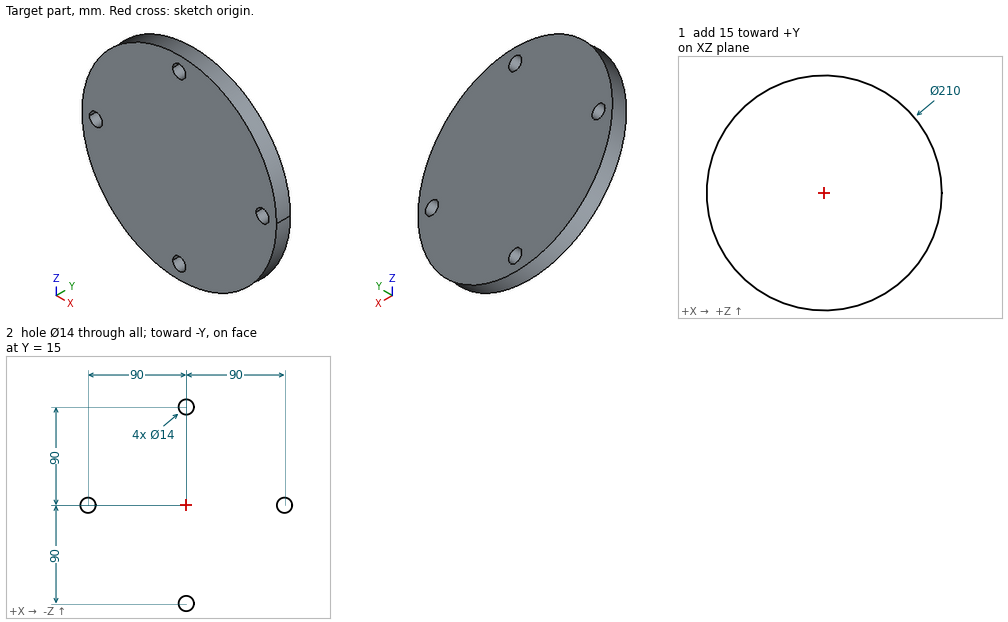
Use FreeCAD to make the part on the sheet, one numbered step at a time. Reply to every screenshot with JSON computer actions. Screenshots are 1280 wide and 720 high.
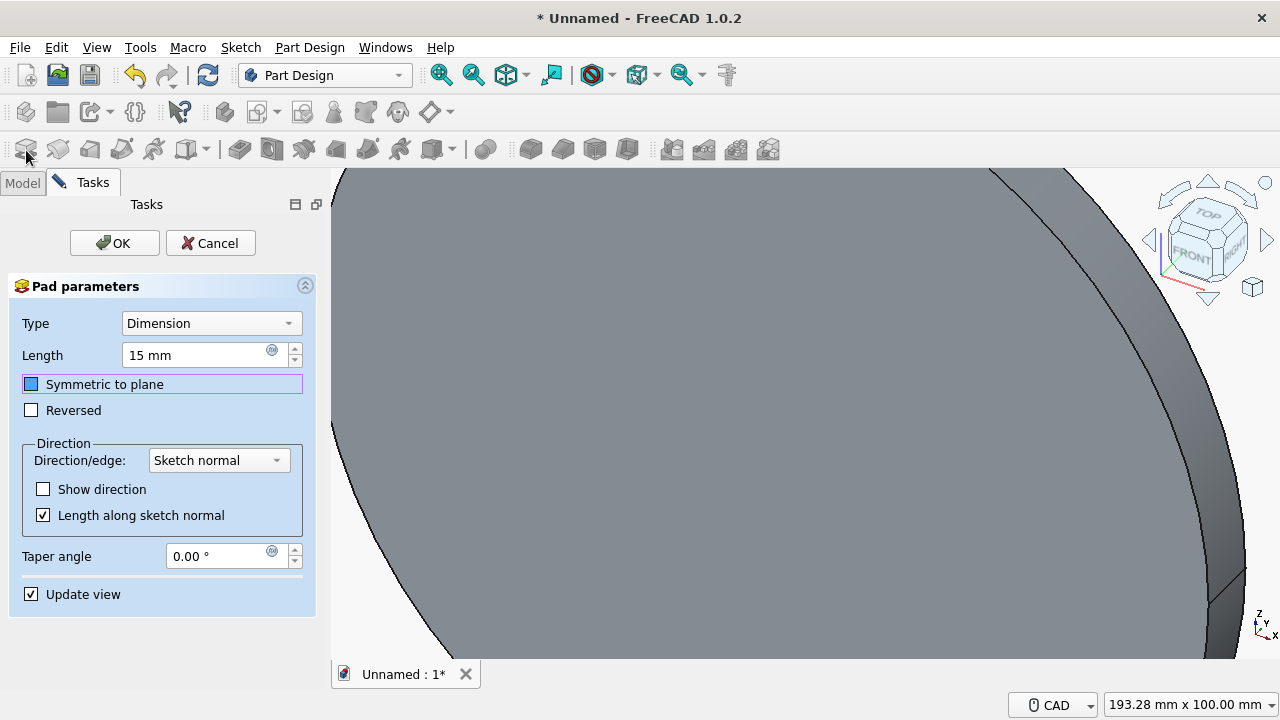
{"action": "left_click", "coordinate": [30, 410]}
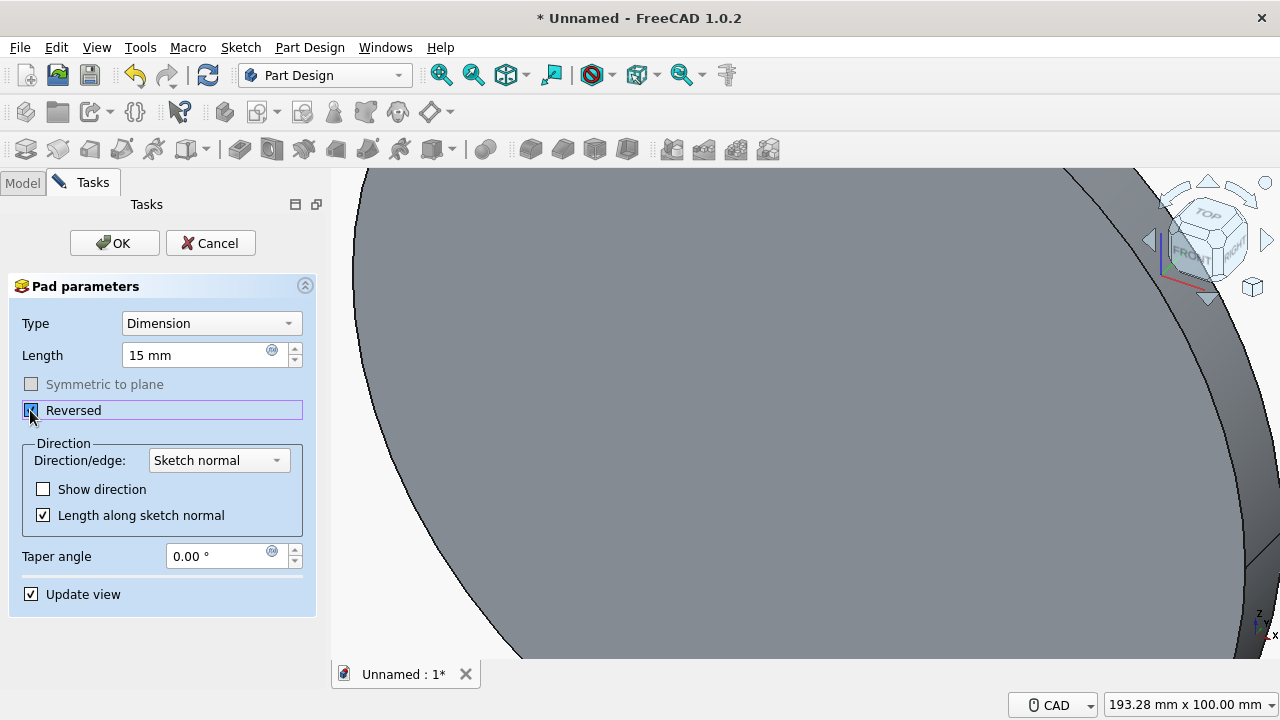
{"action": "left_click", "coordinate": [115, 243]}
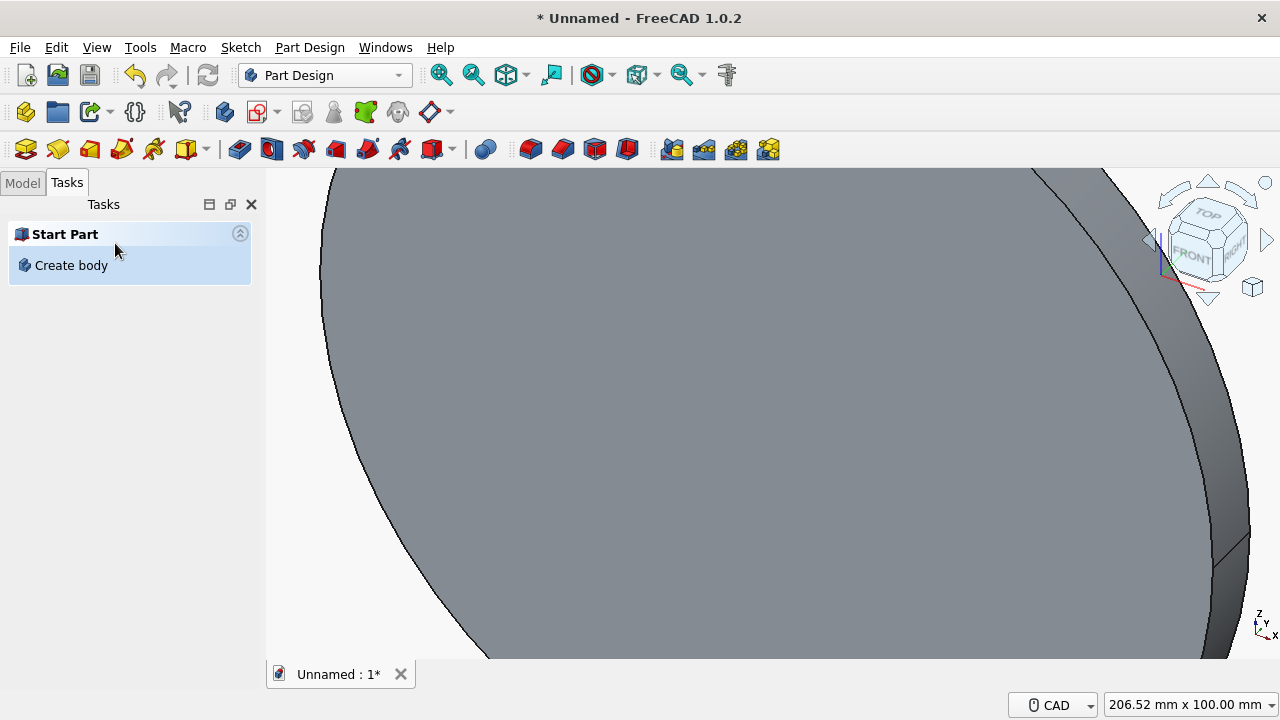
{"action": "left_click", "coordinate": [442, 76]}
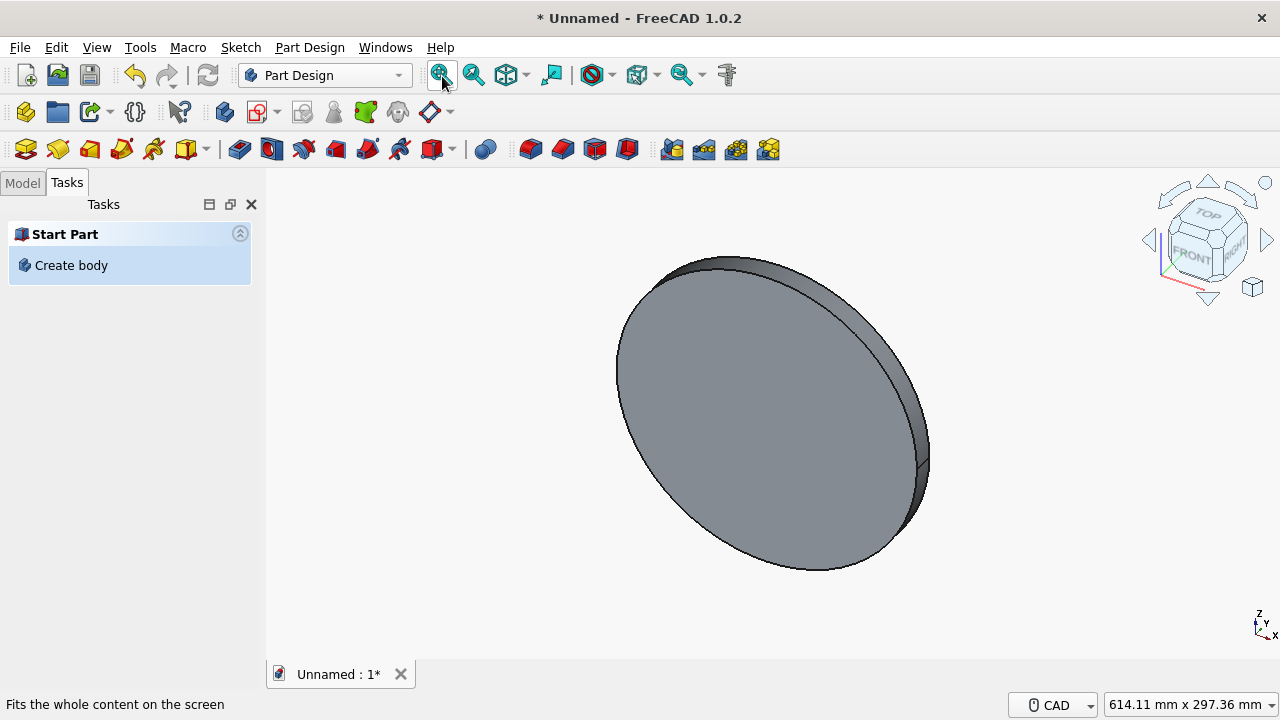
{"action": "key", "text": "4"}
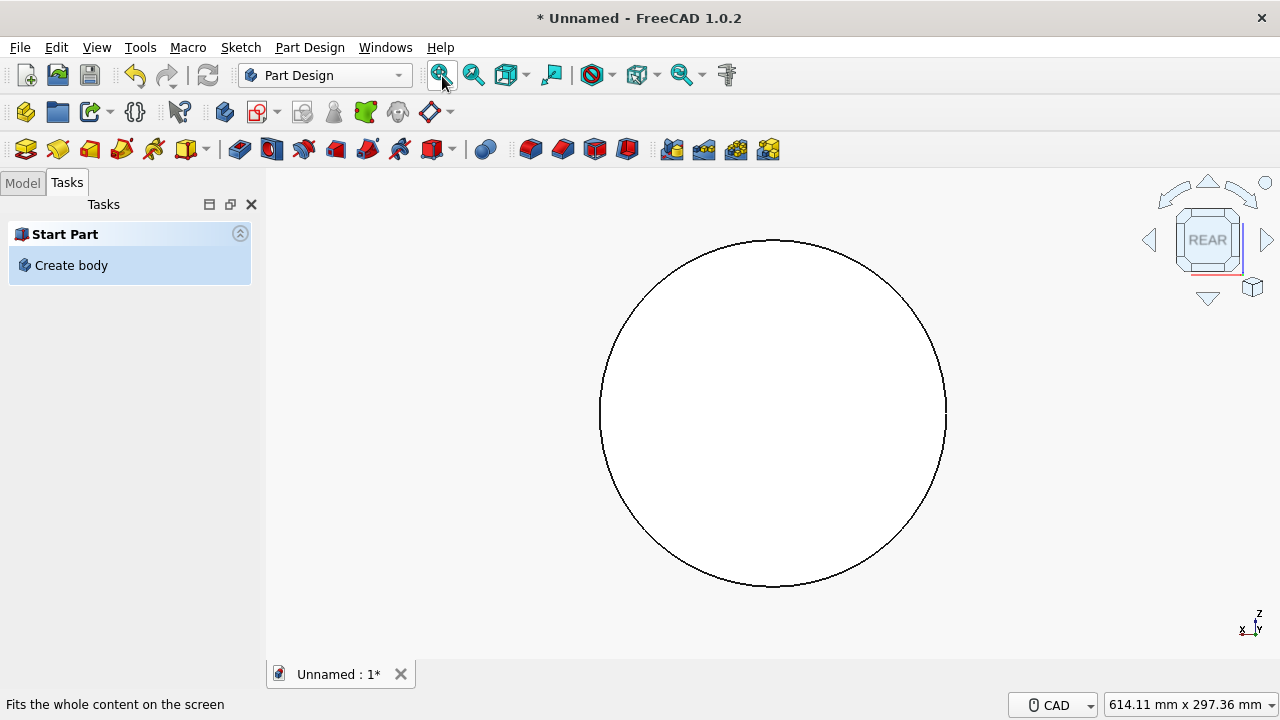
{"action": "left_click", "coordinate": [773, 412]}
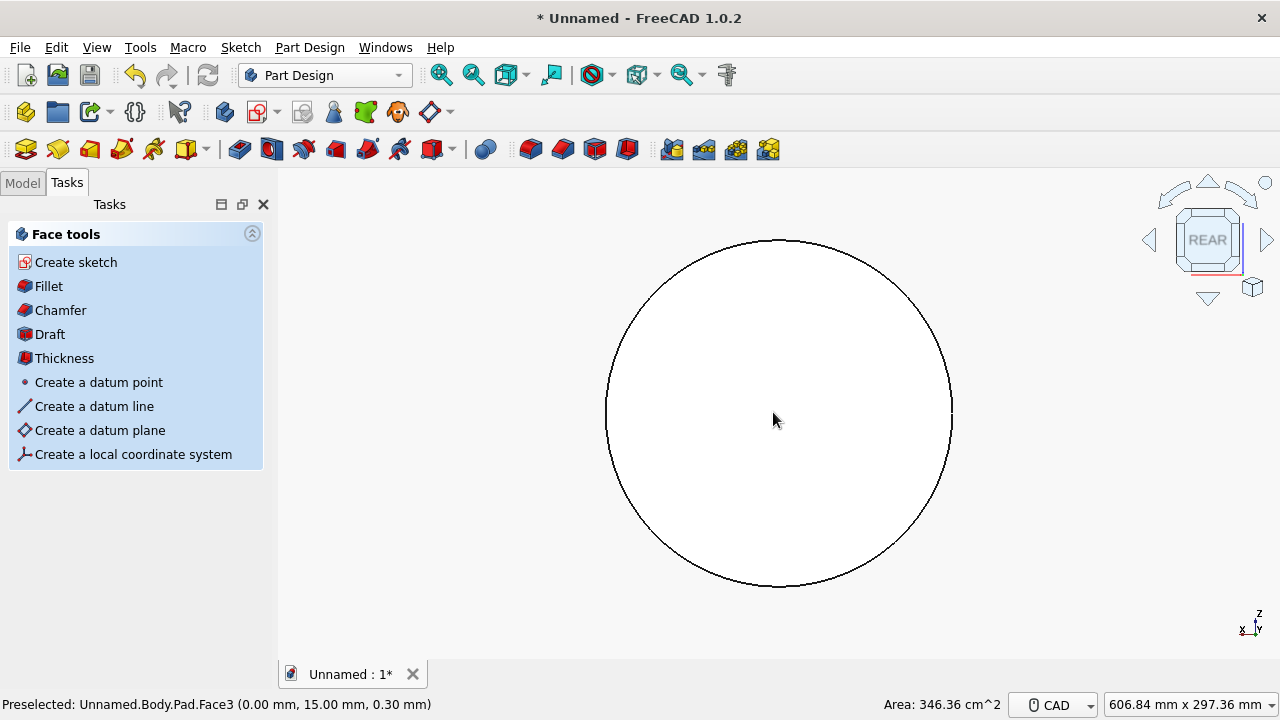
{"action": "left_click", "coordinate": [258, 112]}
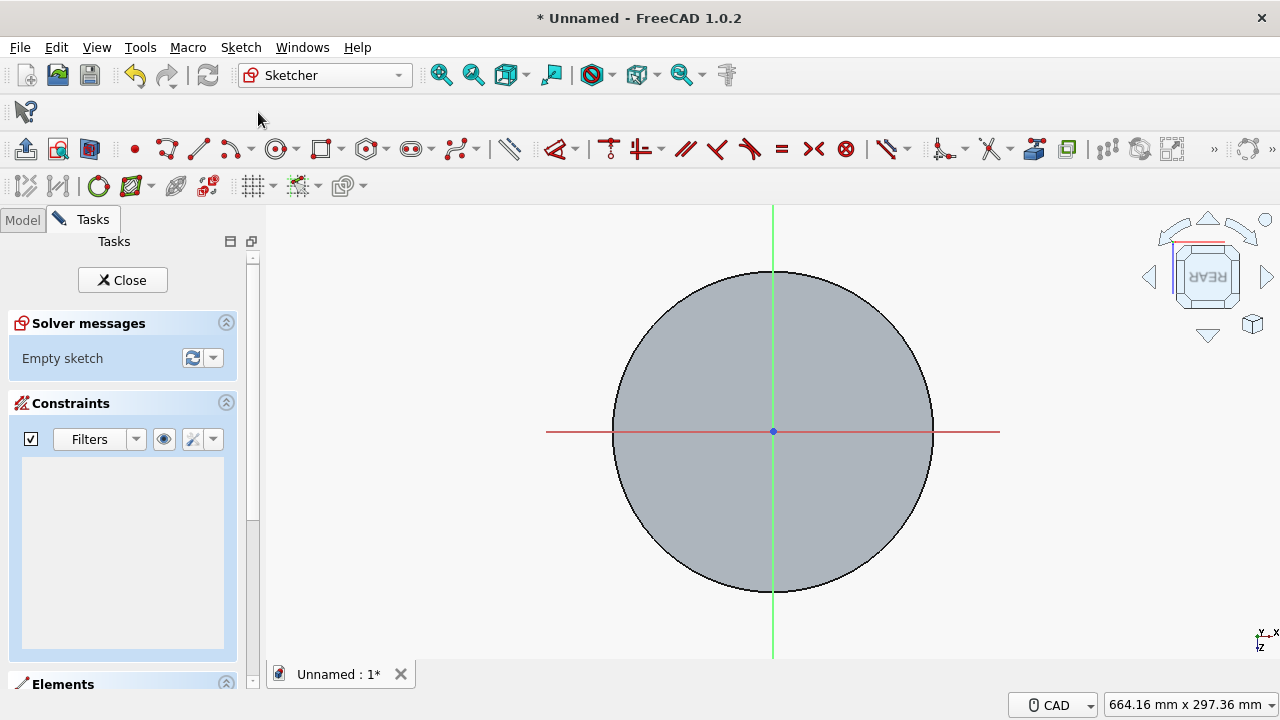
{"action": "left_click", "coordinate": [276, 150]}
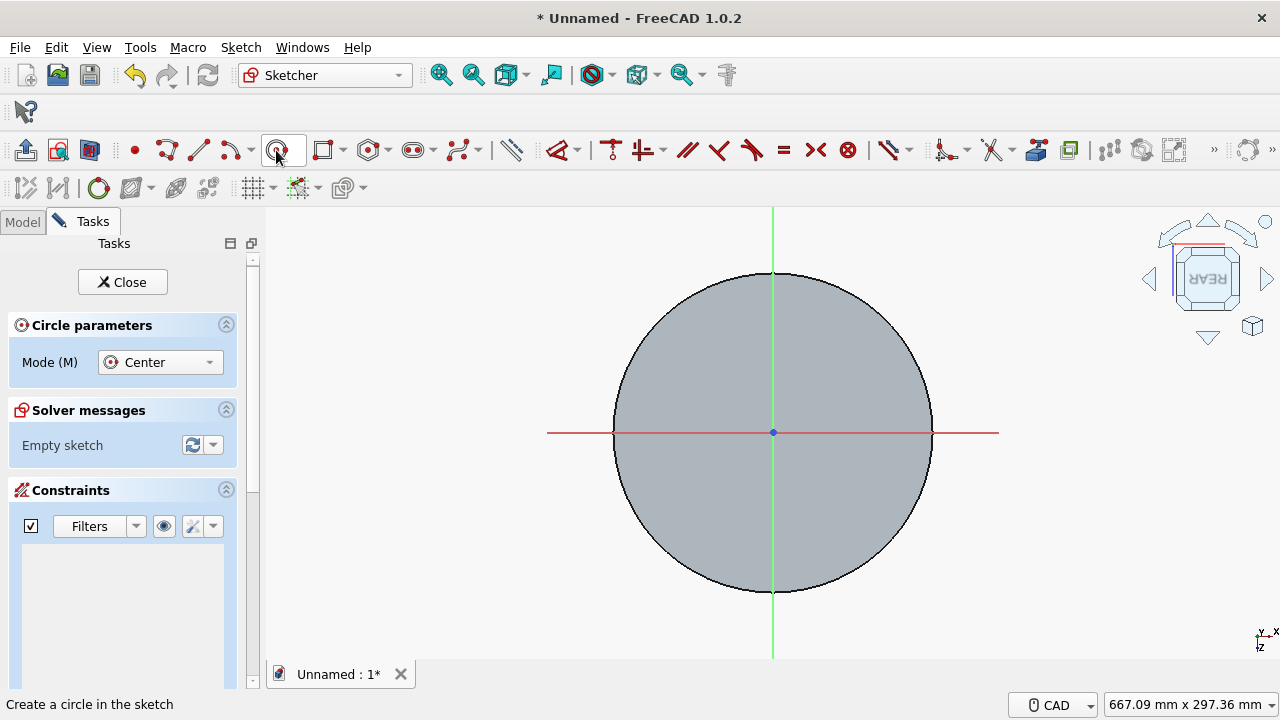
{"action": "scroll", "coordinate": [773, 296], "scroll_direction": "up", "scroll_amount": 4}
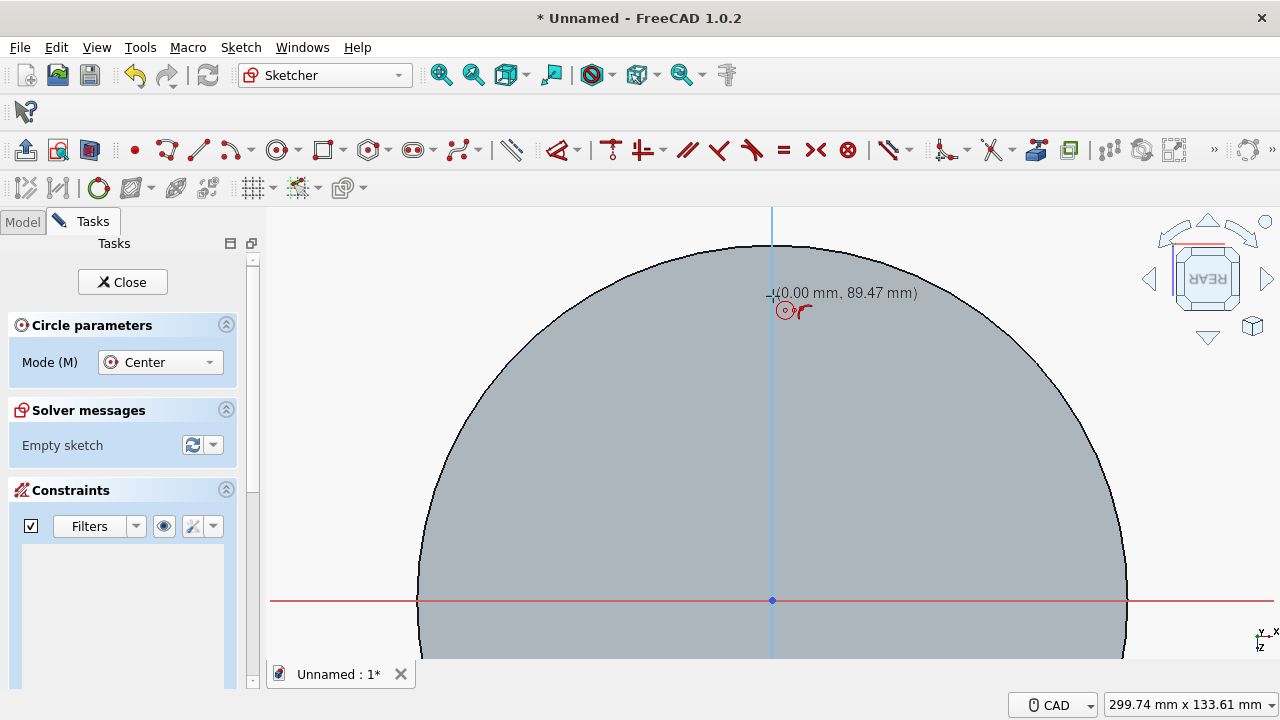
{"action": "left_click", "coordinate": [772, 296]}
{"action": "mouse_move", "coordinate": [789, 279]}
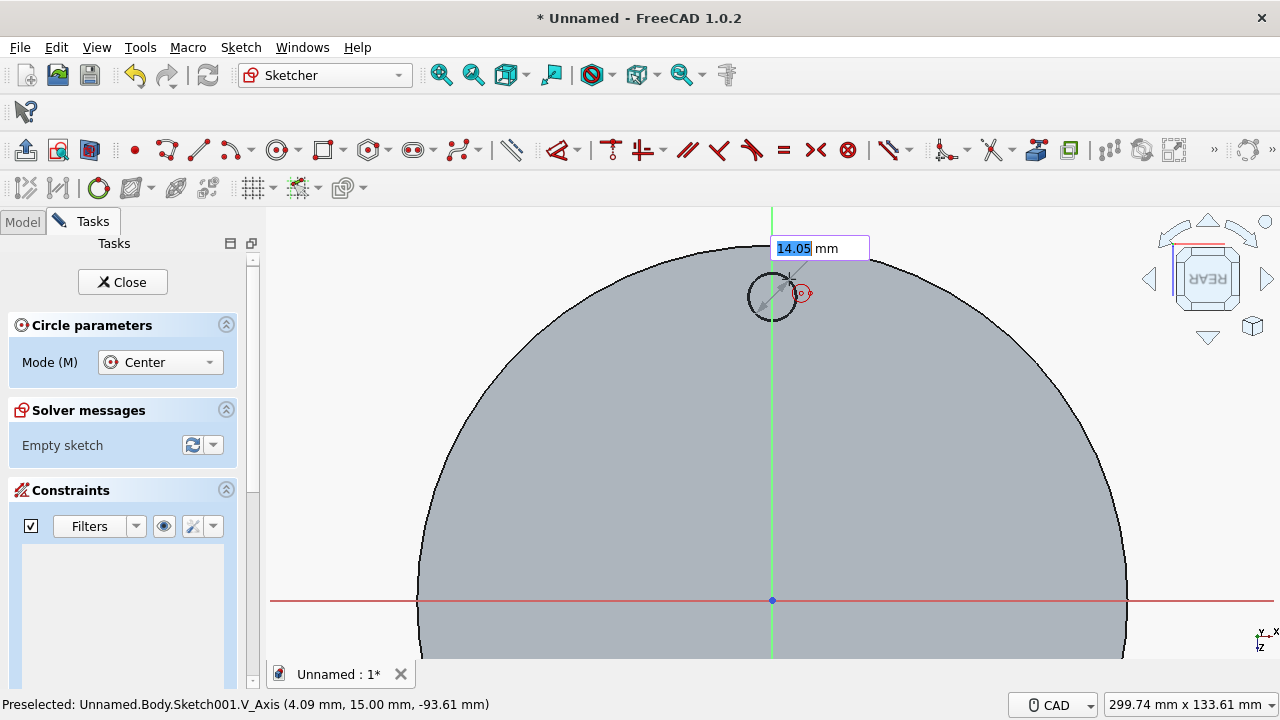
{"action": "type", "text": "14"}
{"action": "key", "text": "Return"}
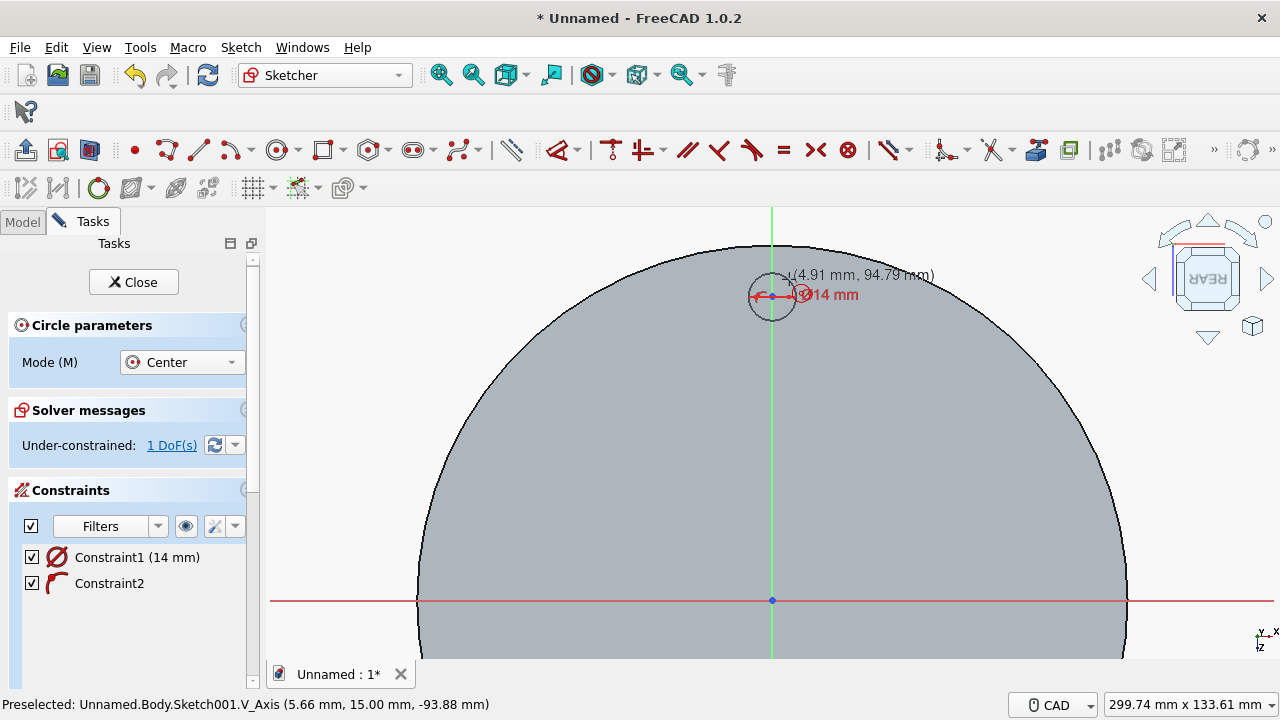
{"action": "left_click", "coordinate": [1077, 601]}
{"action": "mouse_move", "coordinate": [1094, 584]}